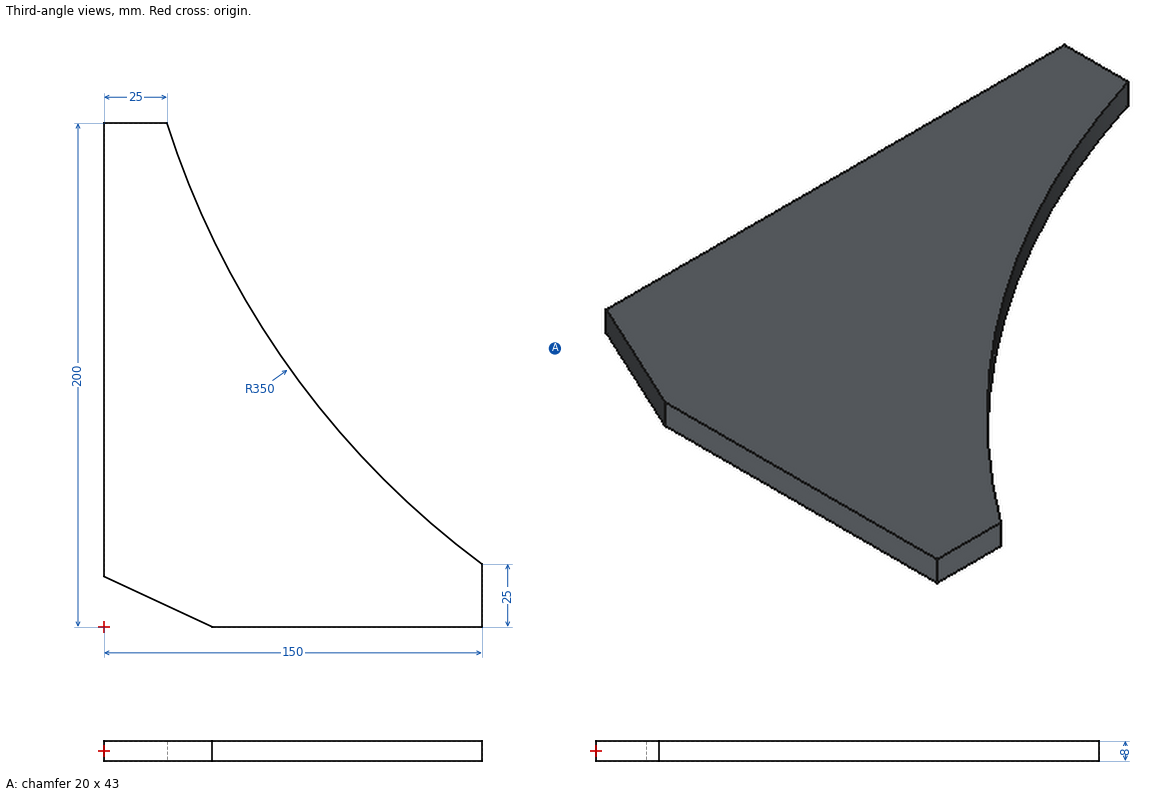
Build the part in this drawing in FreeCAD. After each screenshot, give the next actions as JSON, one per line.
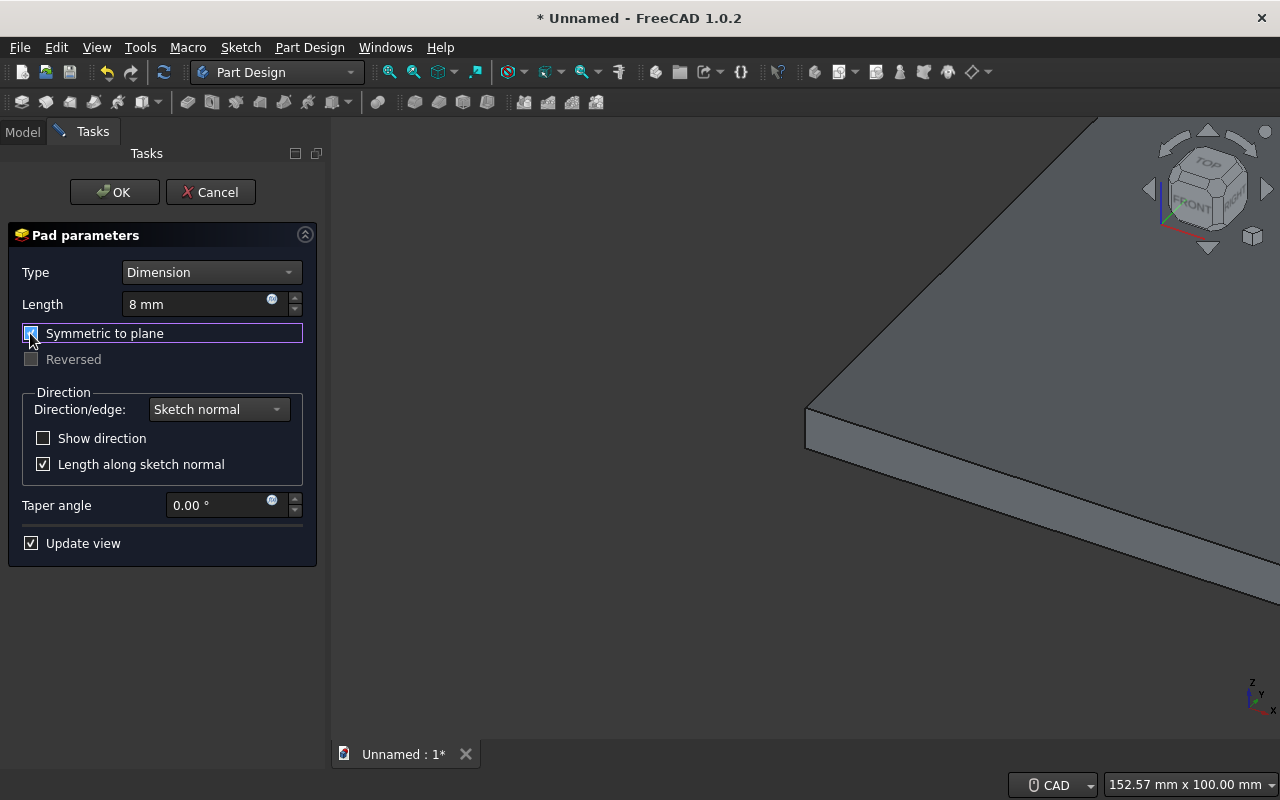
{"action": "left_click", "coordinate": [115, 192]}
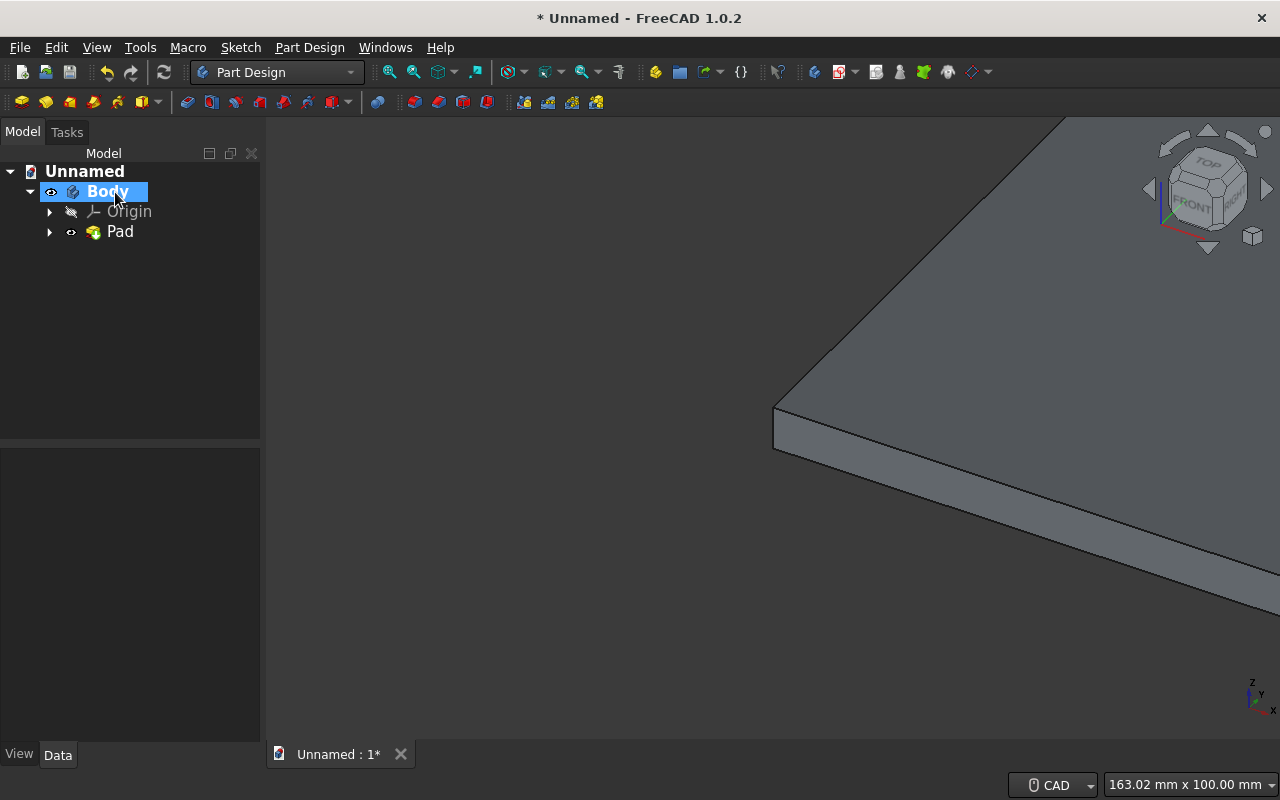
{"action": "key", "text": "v f"}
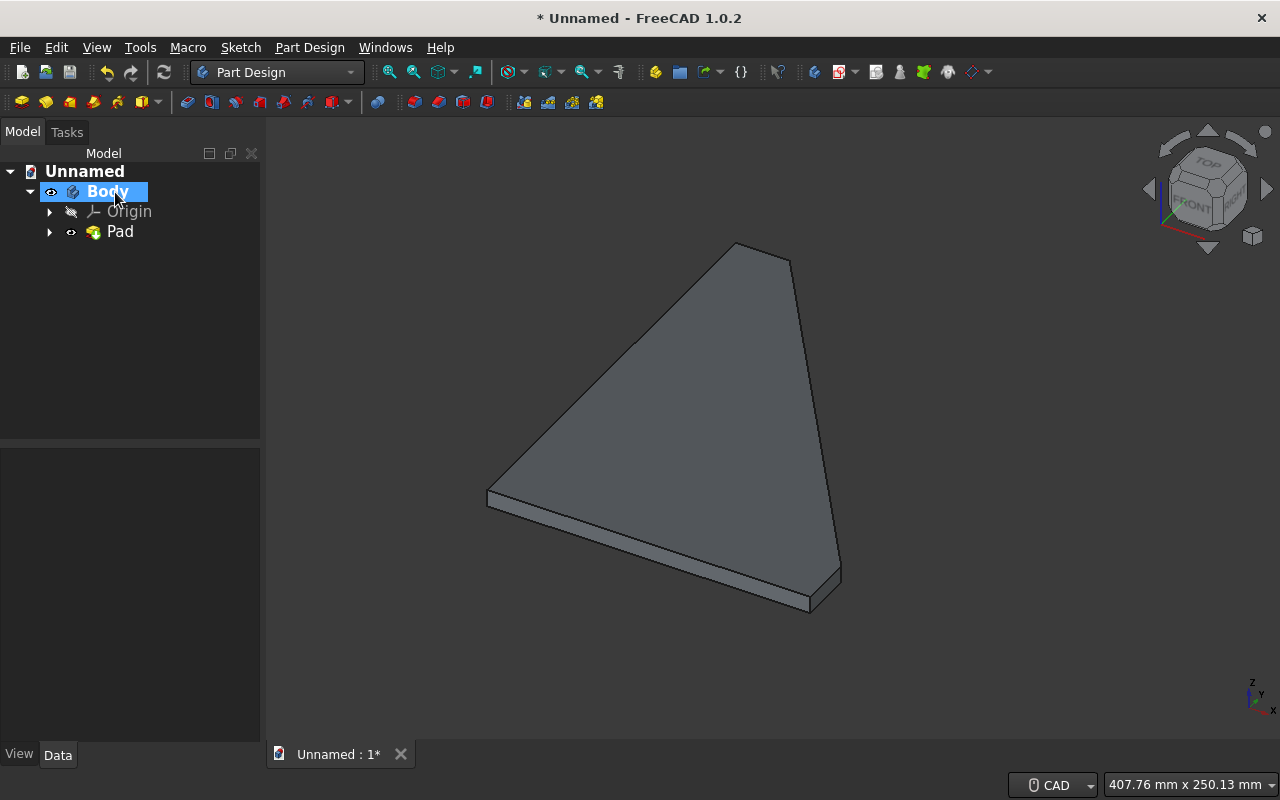
{"action": "scroll", "coordinate": [487, 497], "scroll_direction": "up", "scroll_amount": 4}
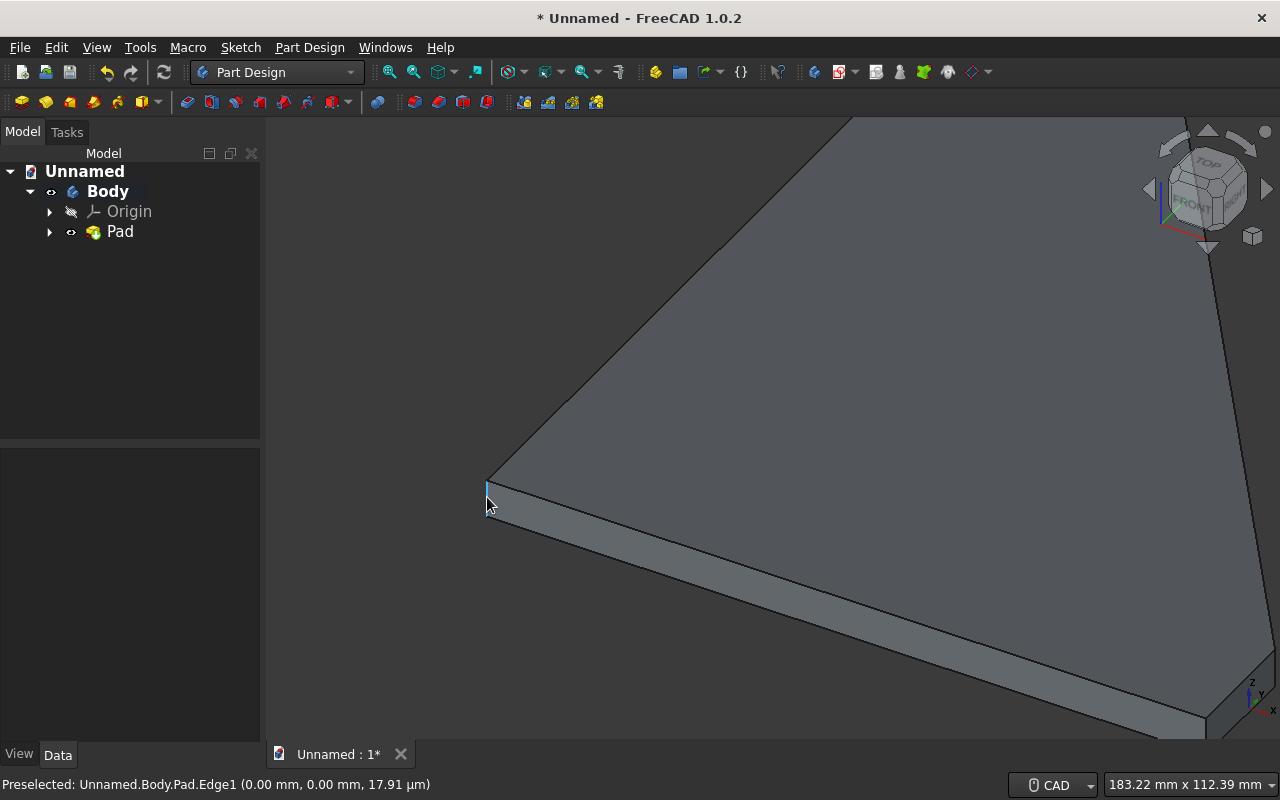
{"action": "key", "text": "v f"}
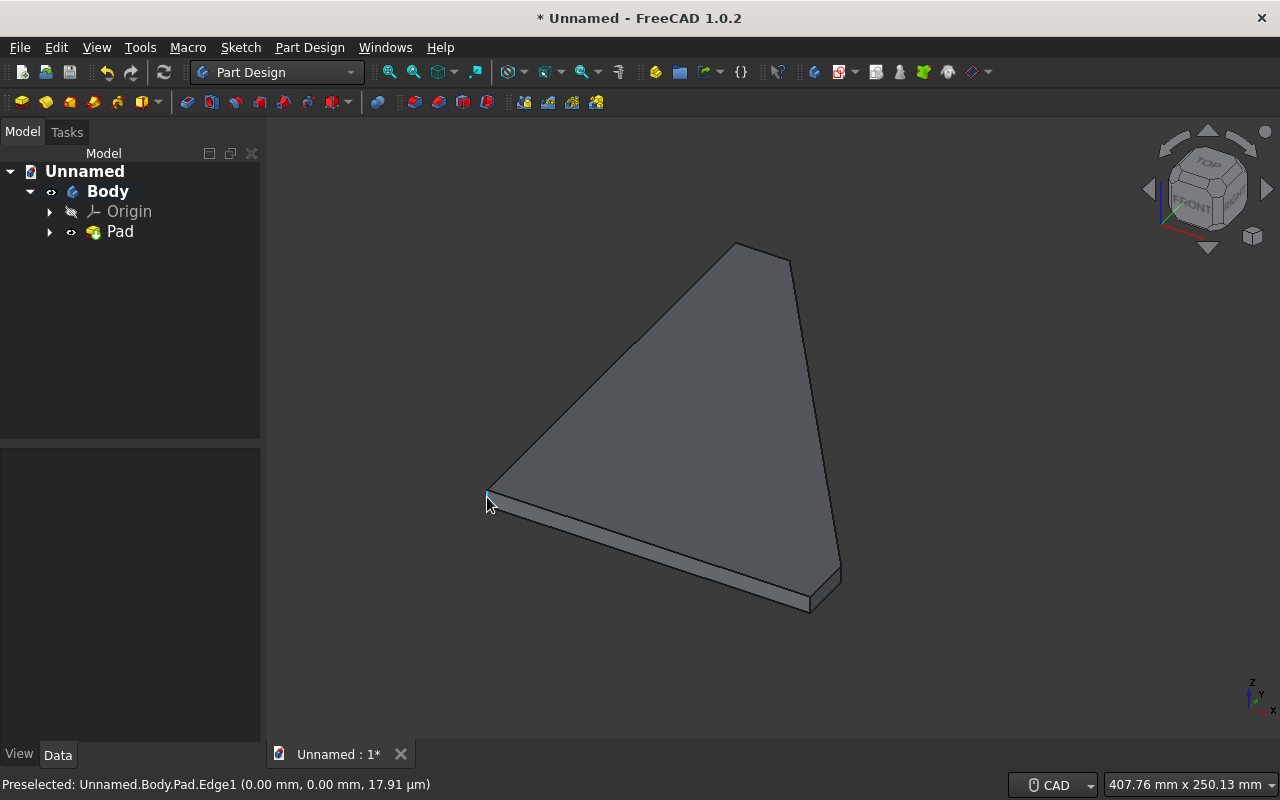
{"action": "key", "text": "0"}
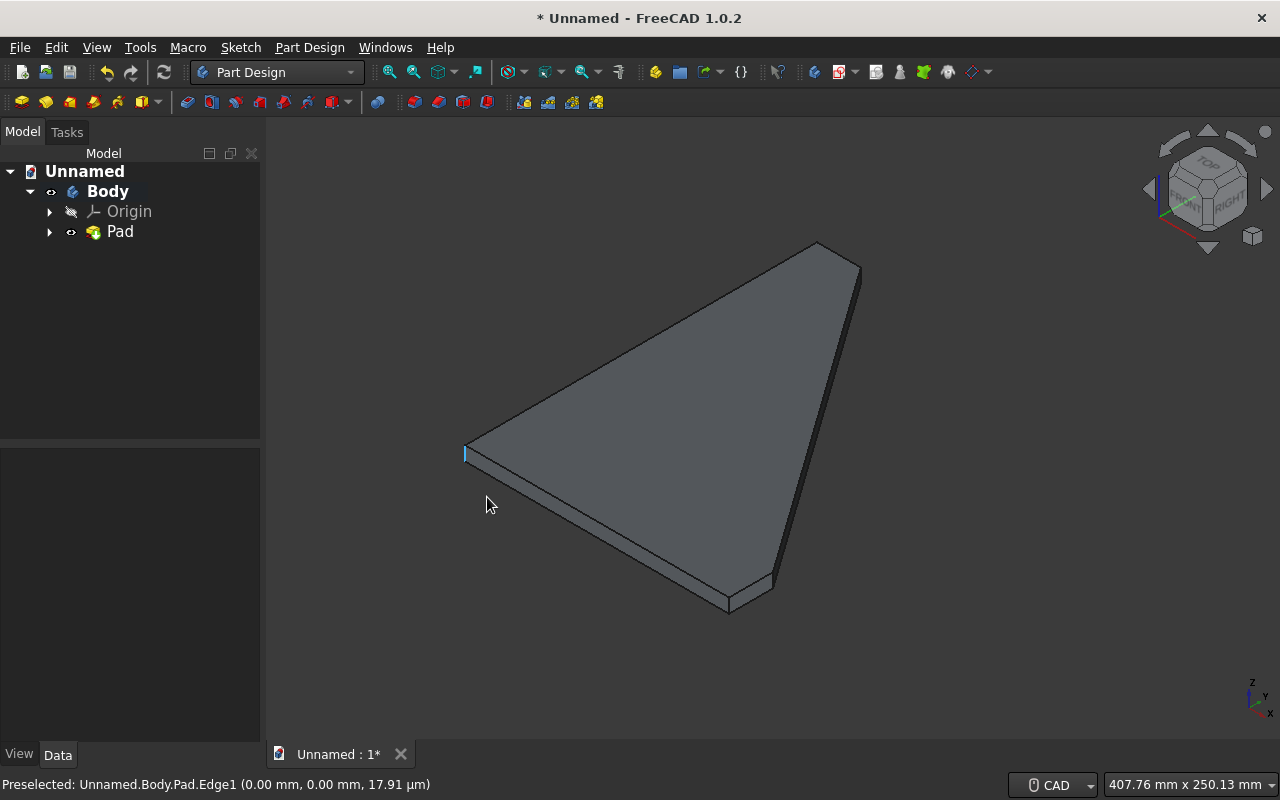
{"action": "scroll", "coordinate": [465, 452], "scroll_direction": "up", "scroll_amount": 4}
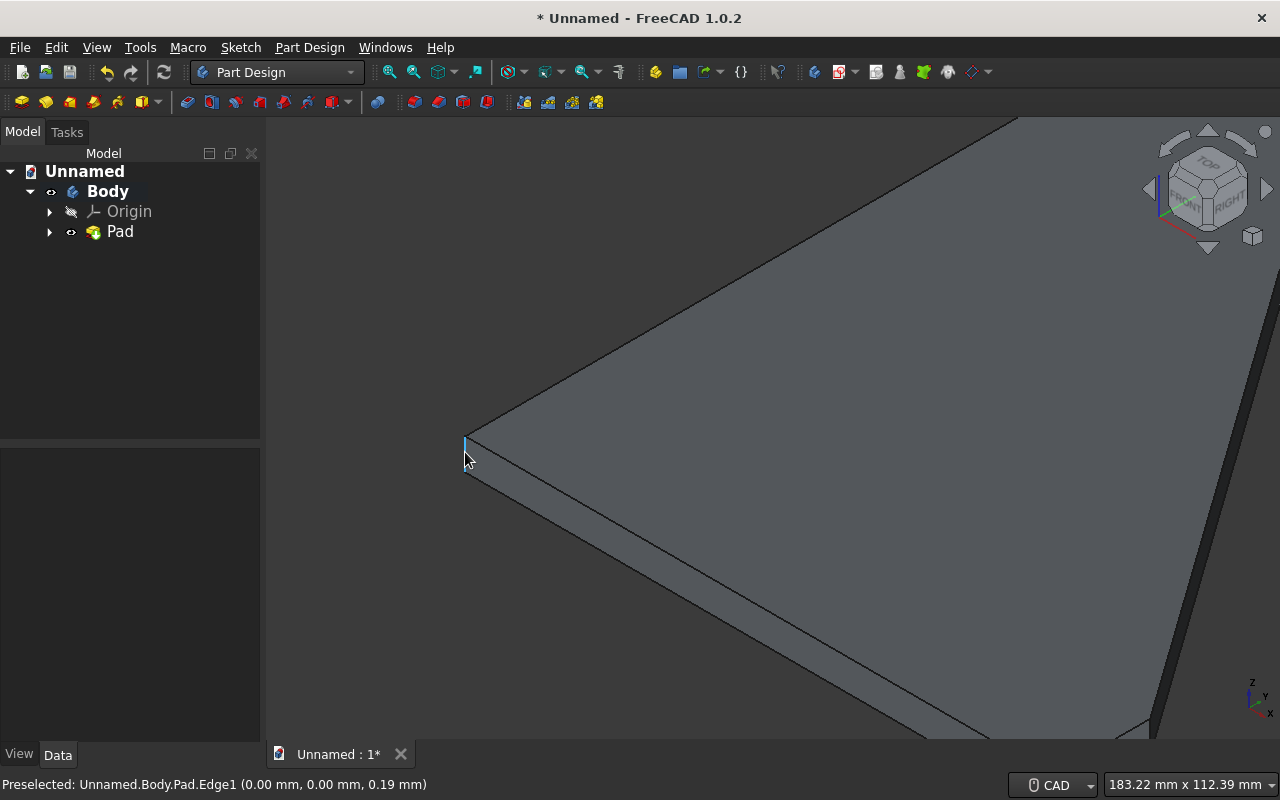
{"action": "key", "text": "v f"}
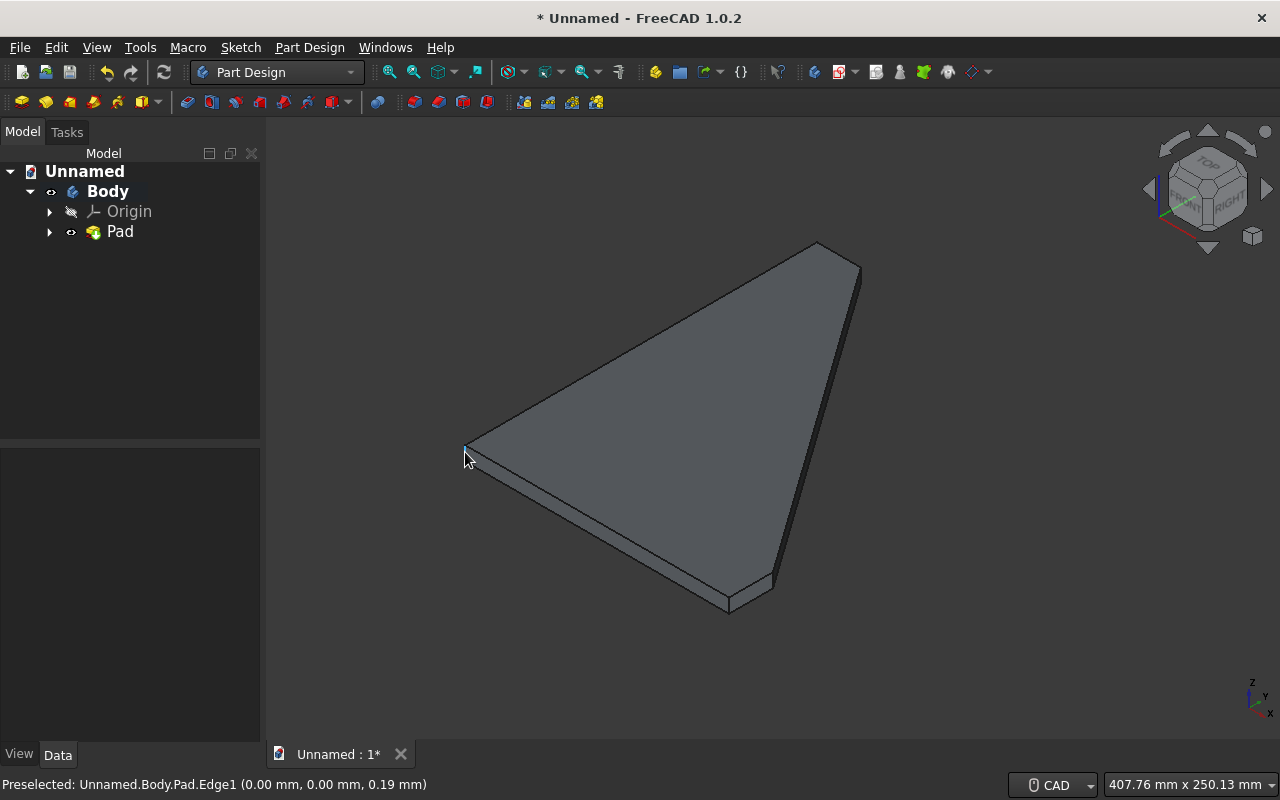
{"action": "key", "text": "2"}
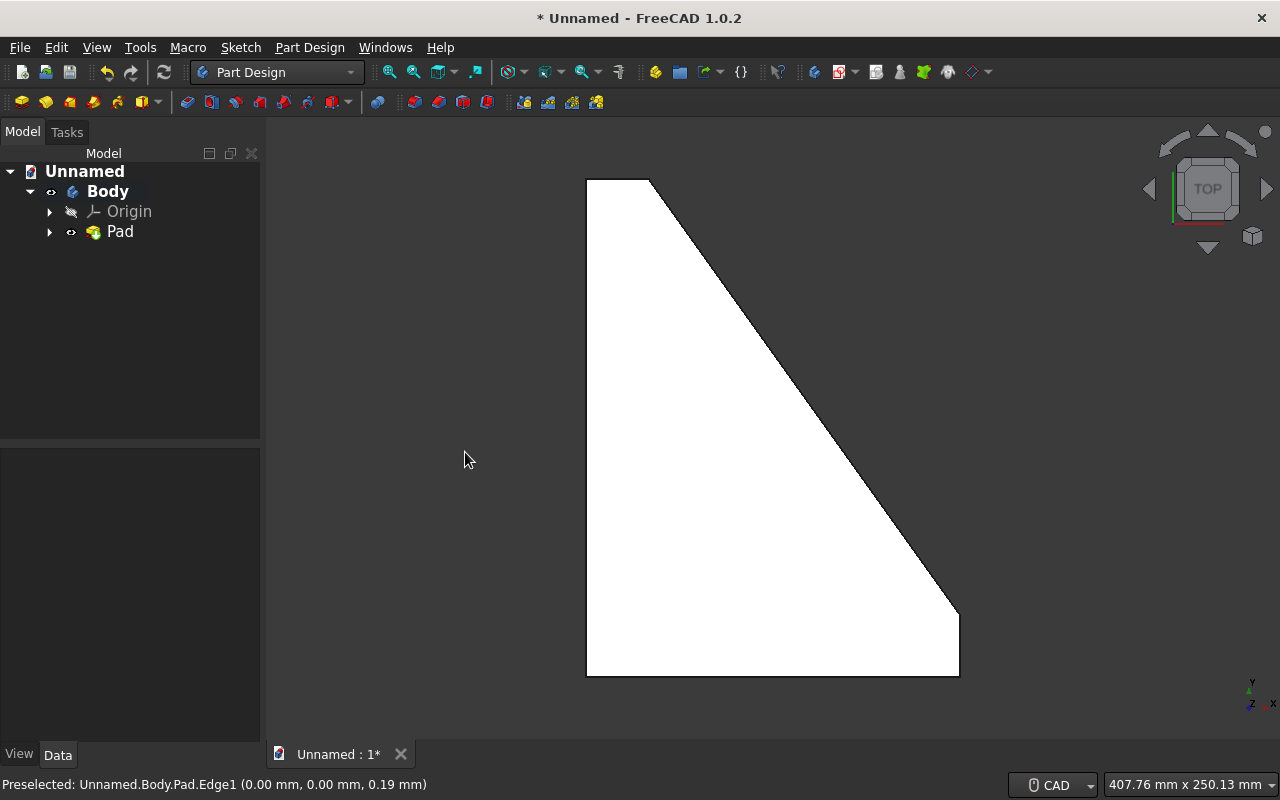
{"action": "scroll", "coordinate": [586, 676], "scroll_direction": "up", "scroll_amount": 4}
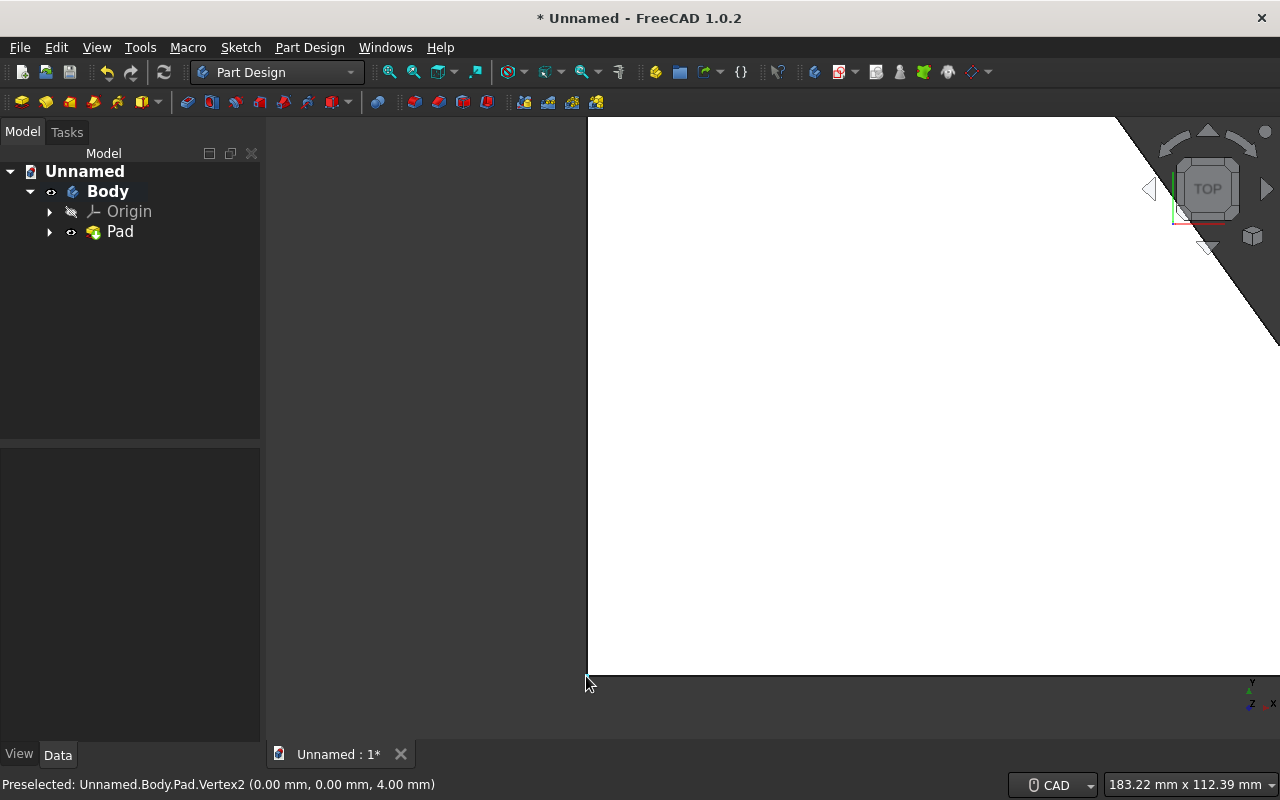
{"action": "key", "text": "v f"}